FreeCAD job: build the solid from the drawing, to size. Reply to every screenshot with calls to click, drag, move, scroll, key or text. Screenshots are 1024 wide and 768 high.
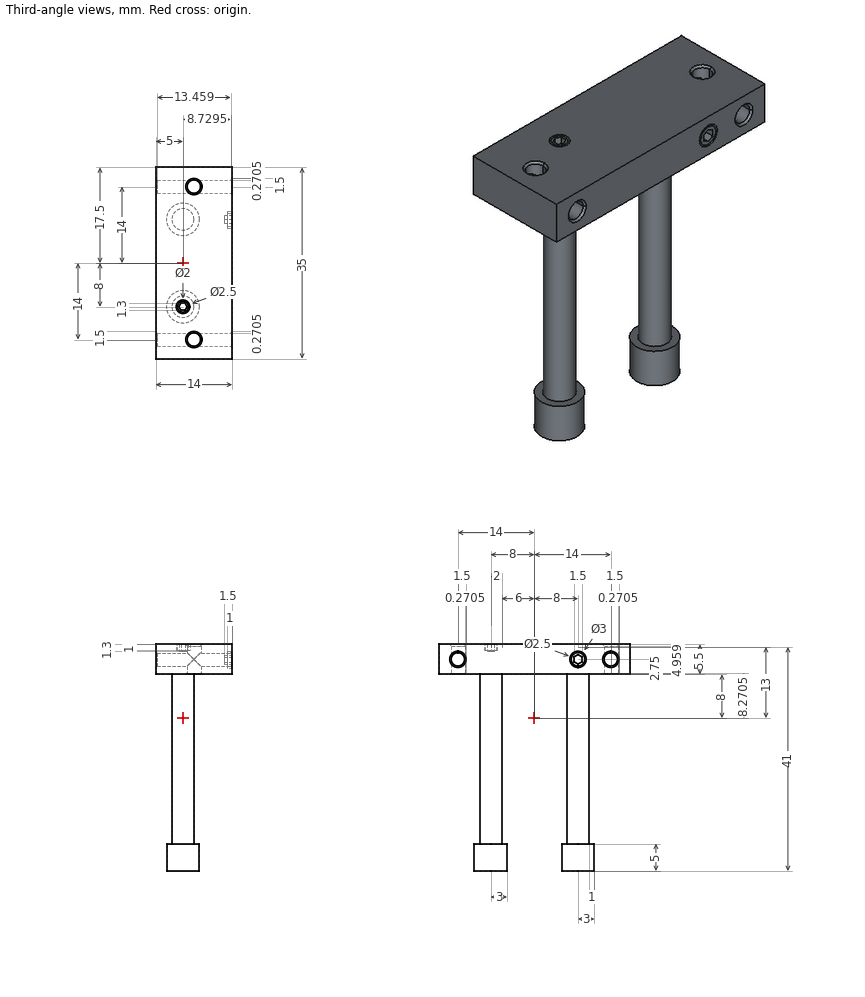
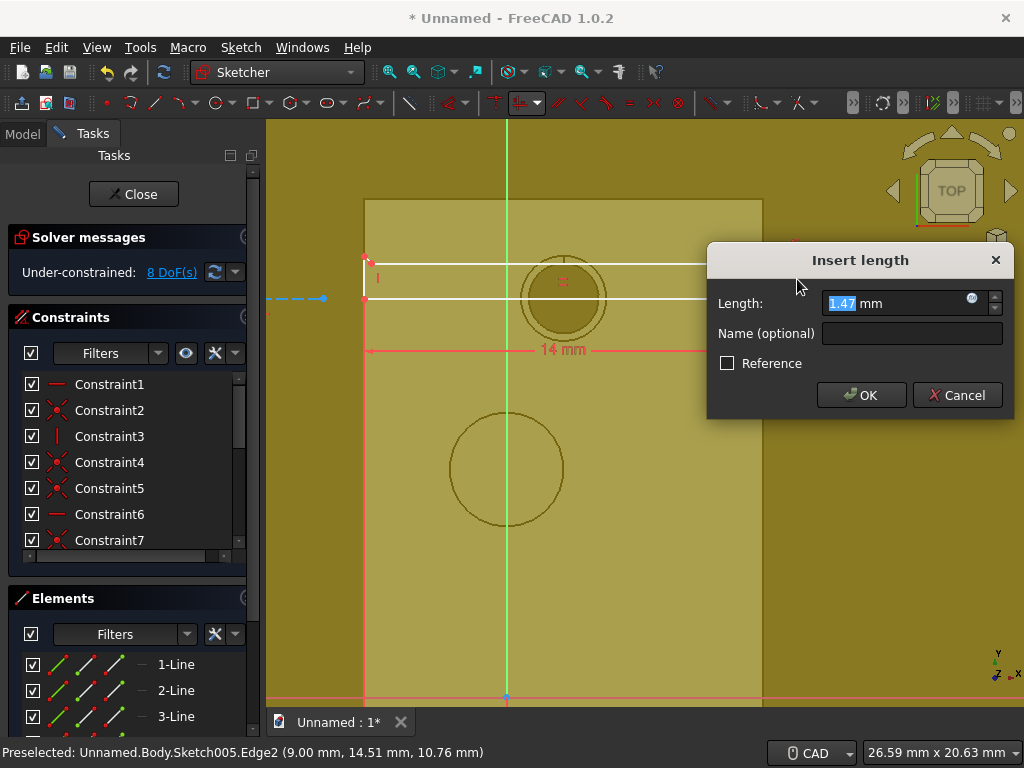
text(1.5)
key(Return)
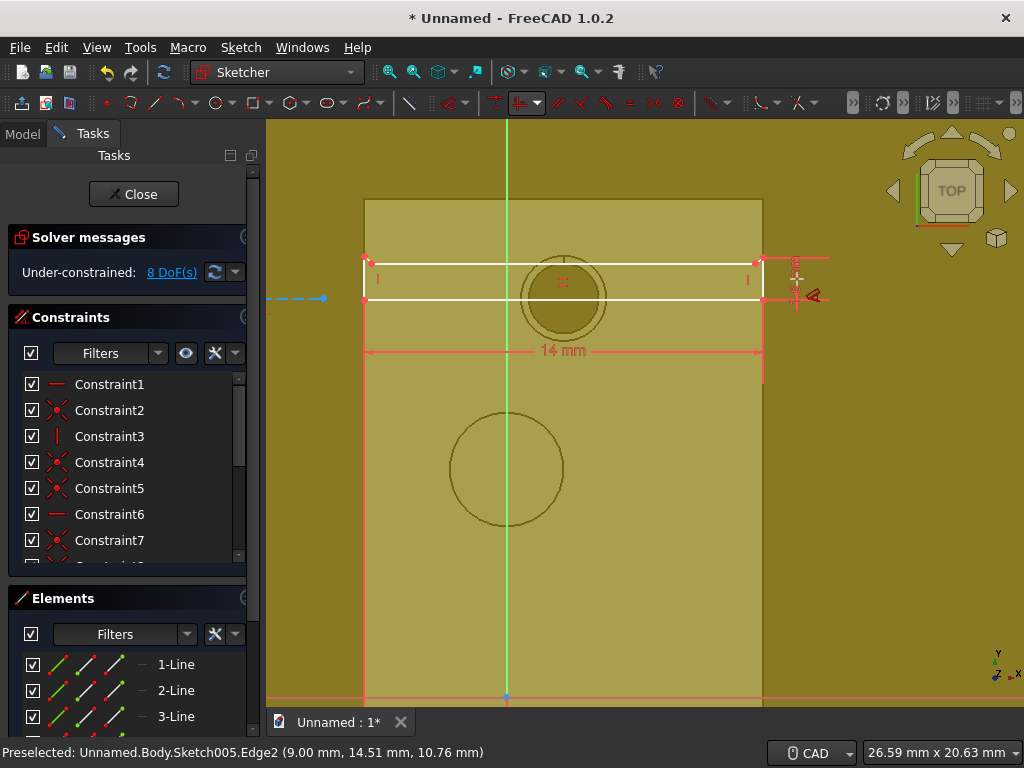
scroll(364, 269, up, 2)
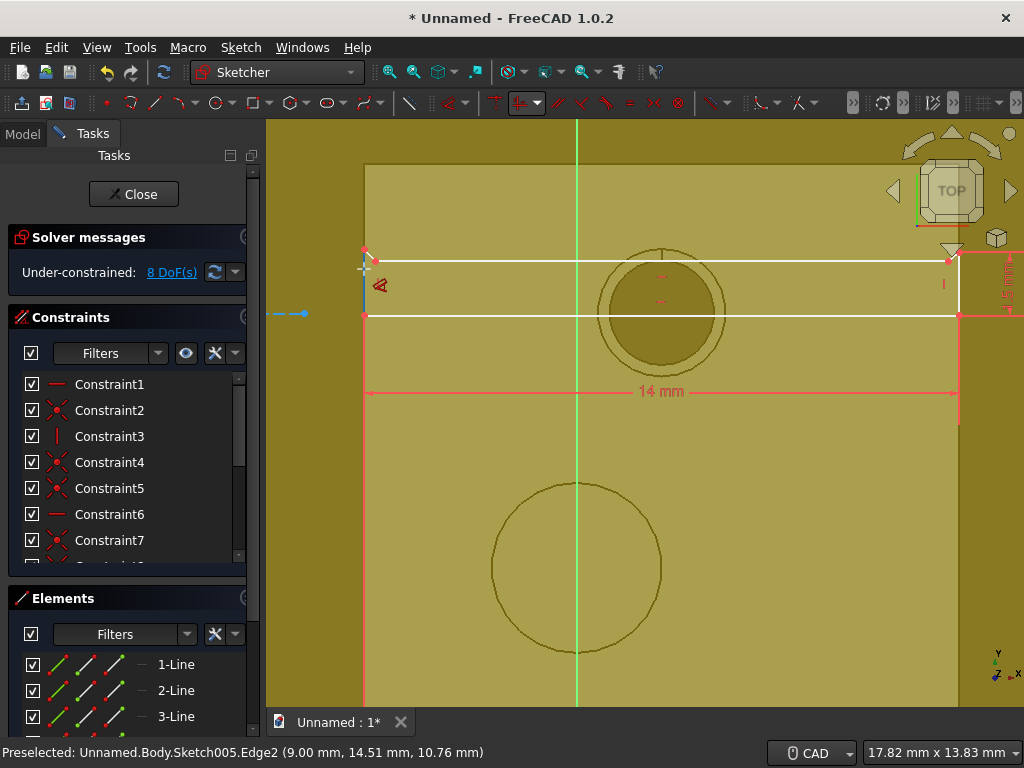
click(364, 269)
click(330, 283)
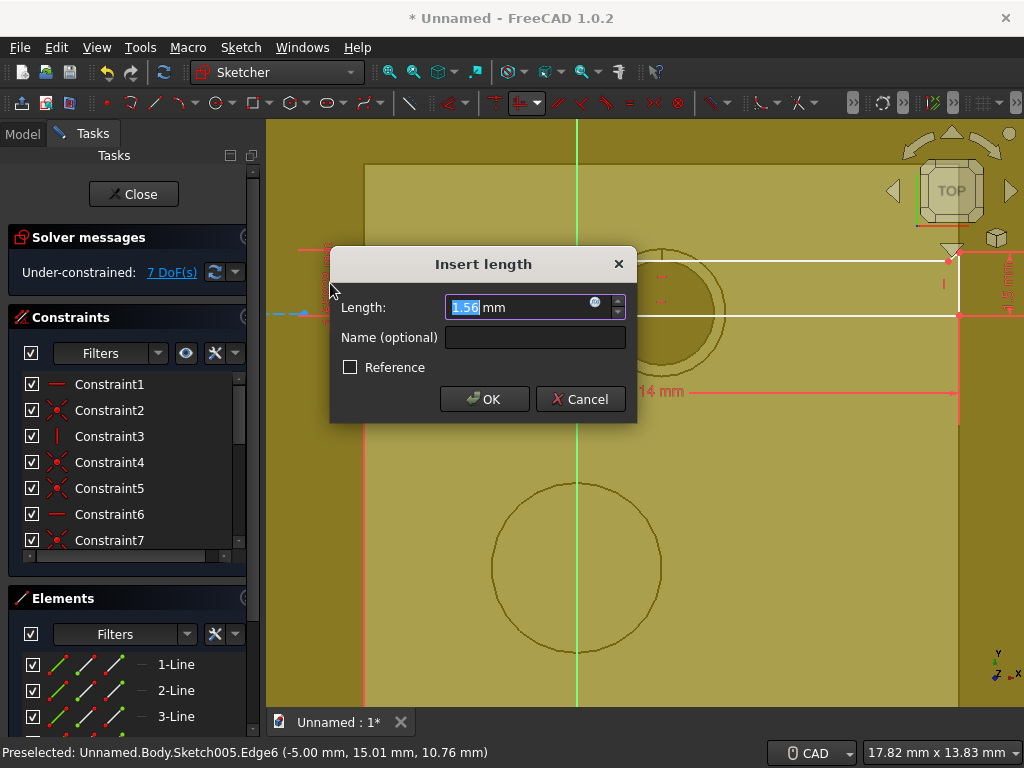
text(1.5)
key(Return)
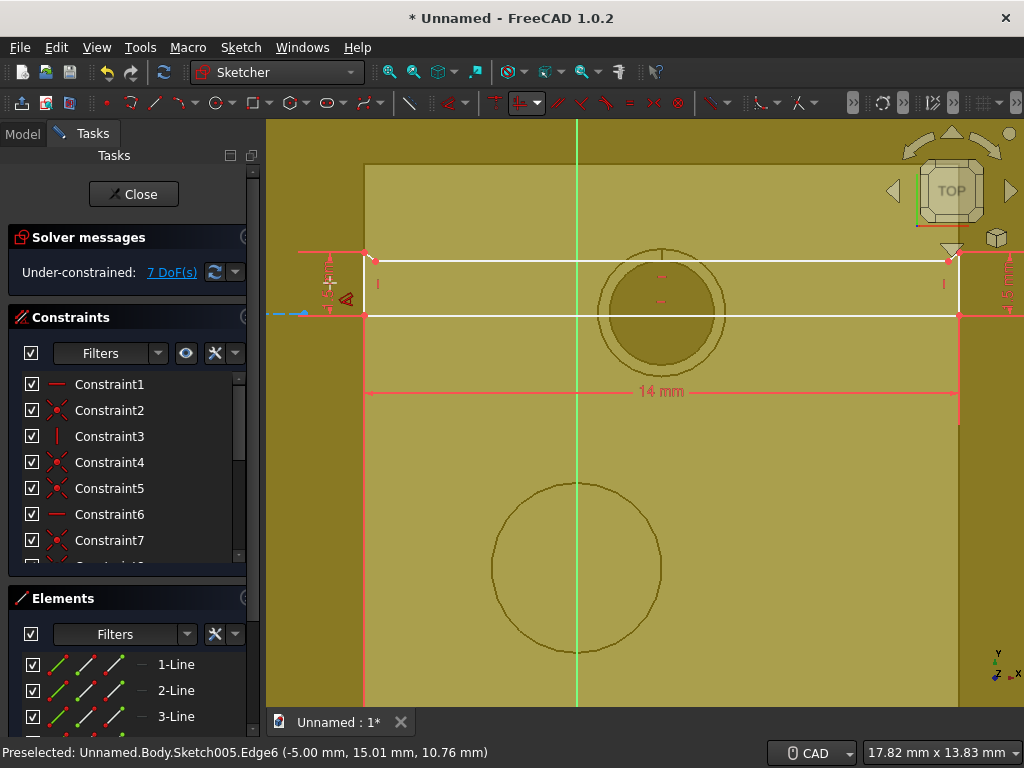
click(364, 316)
click(330, 497)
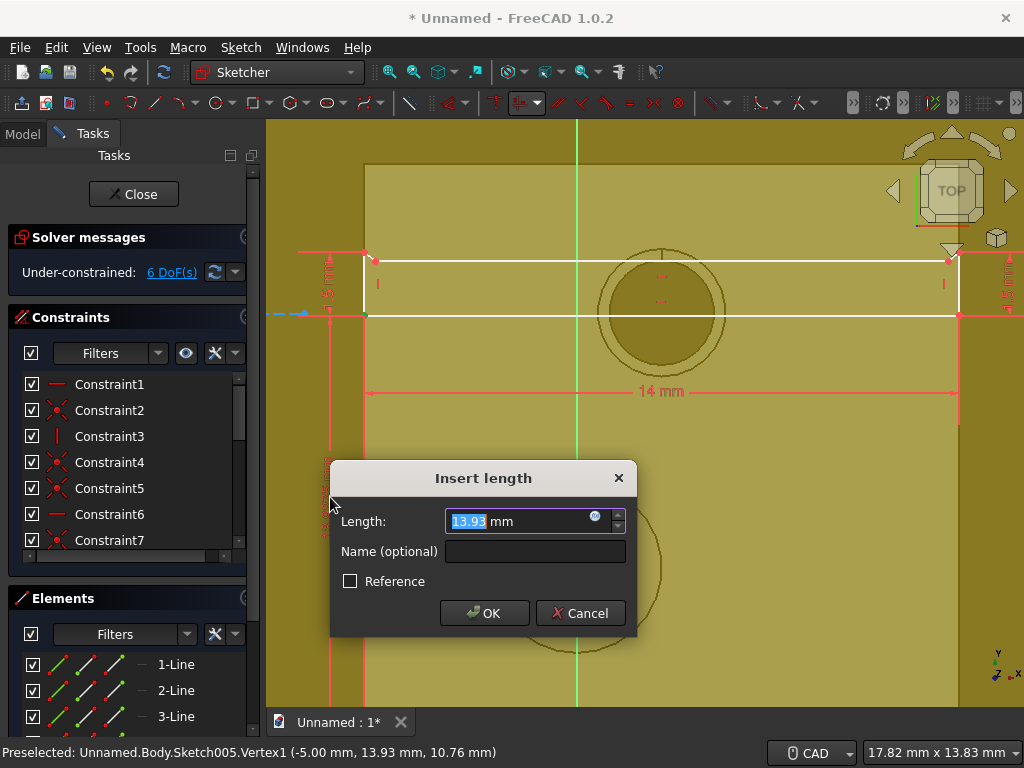
text(14)
key(Return)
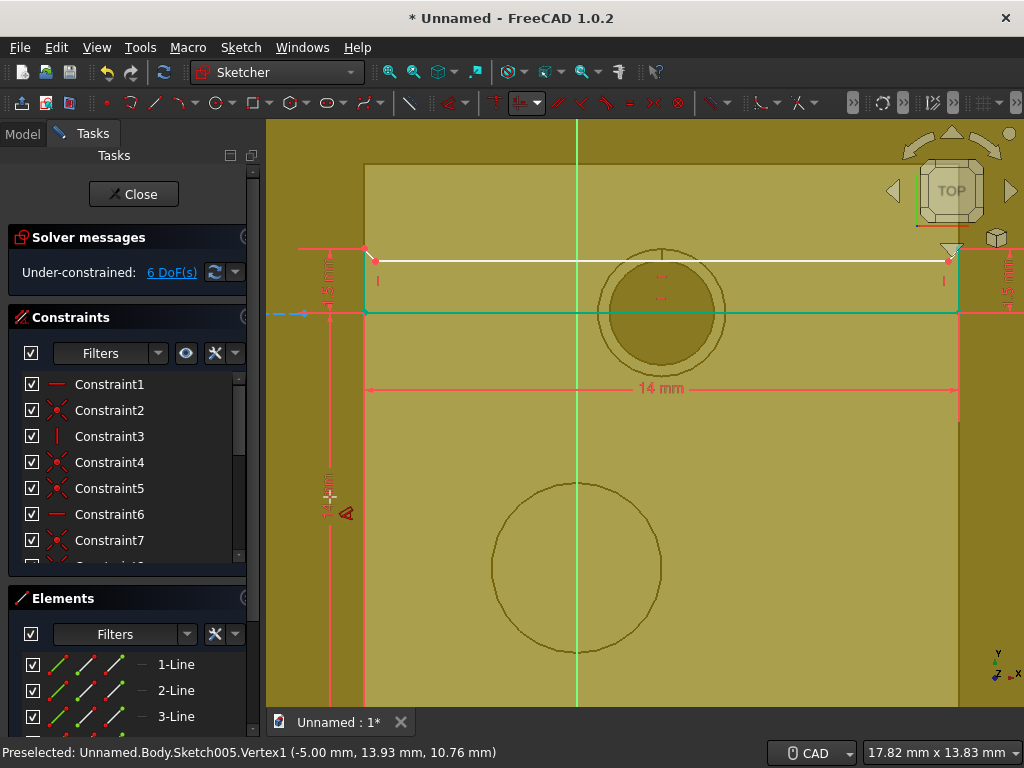
click(304, 314)
click(611, 496)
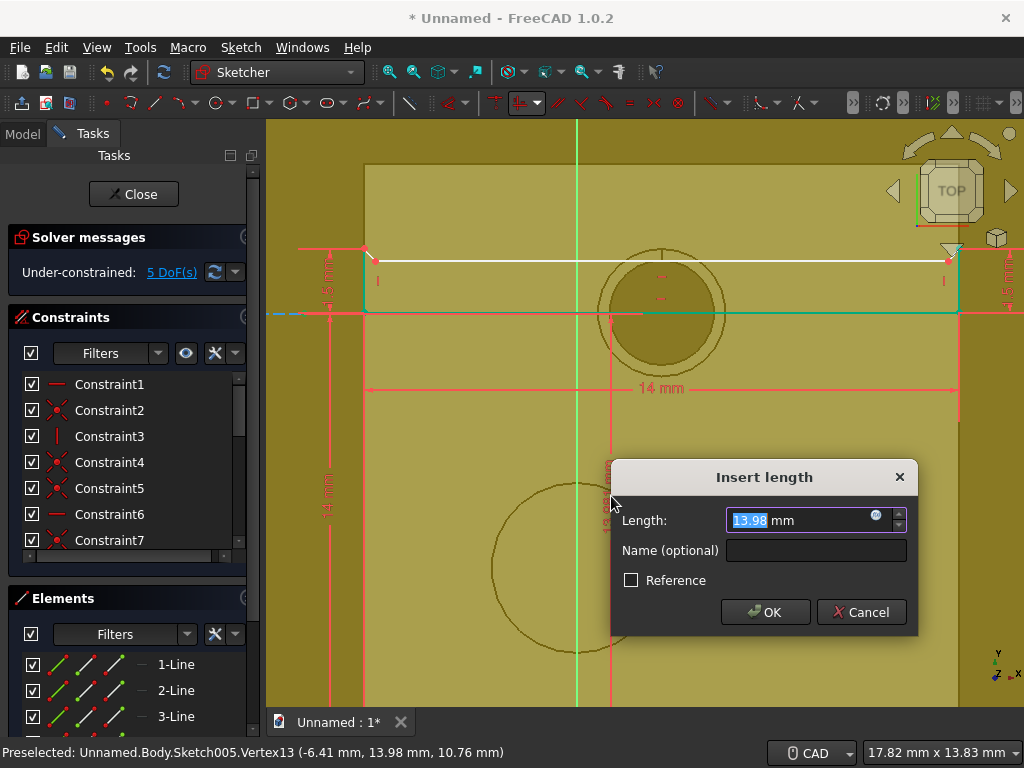
text(14)
key(Return)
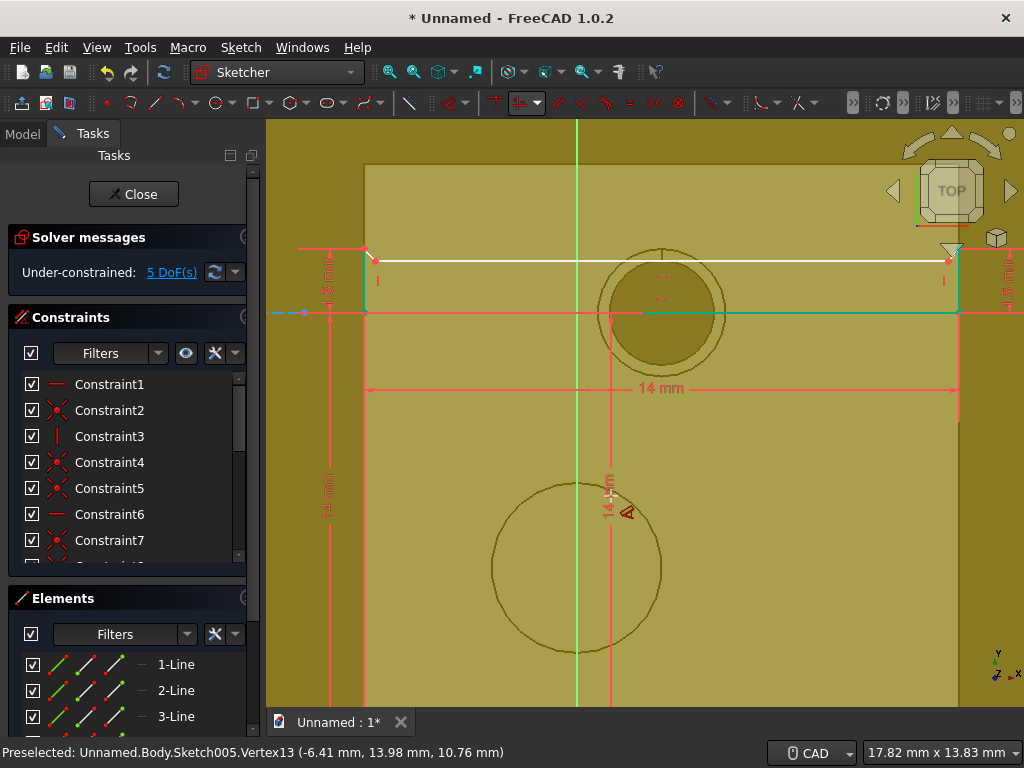
click(776, 261)
click(617, 227)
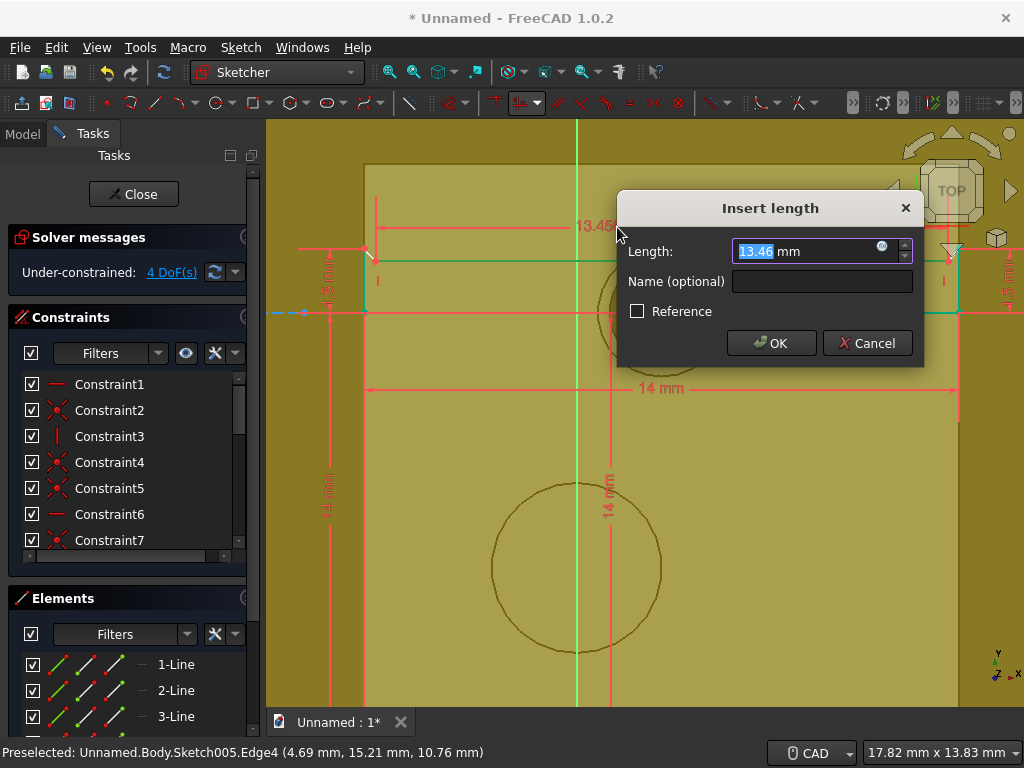
text(13.459)
key(Return)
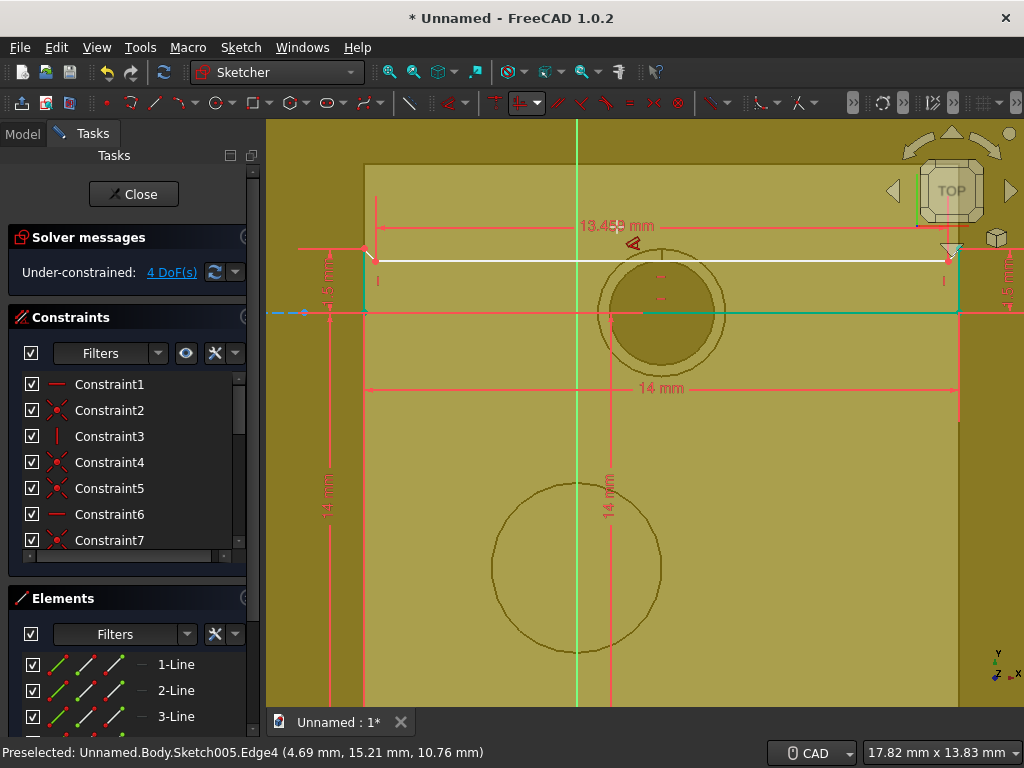
scroll(604, 278, down, 4)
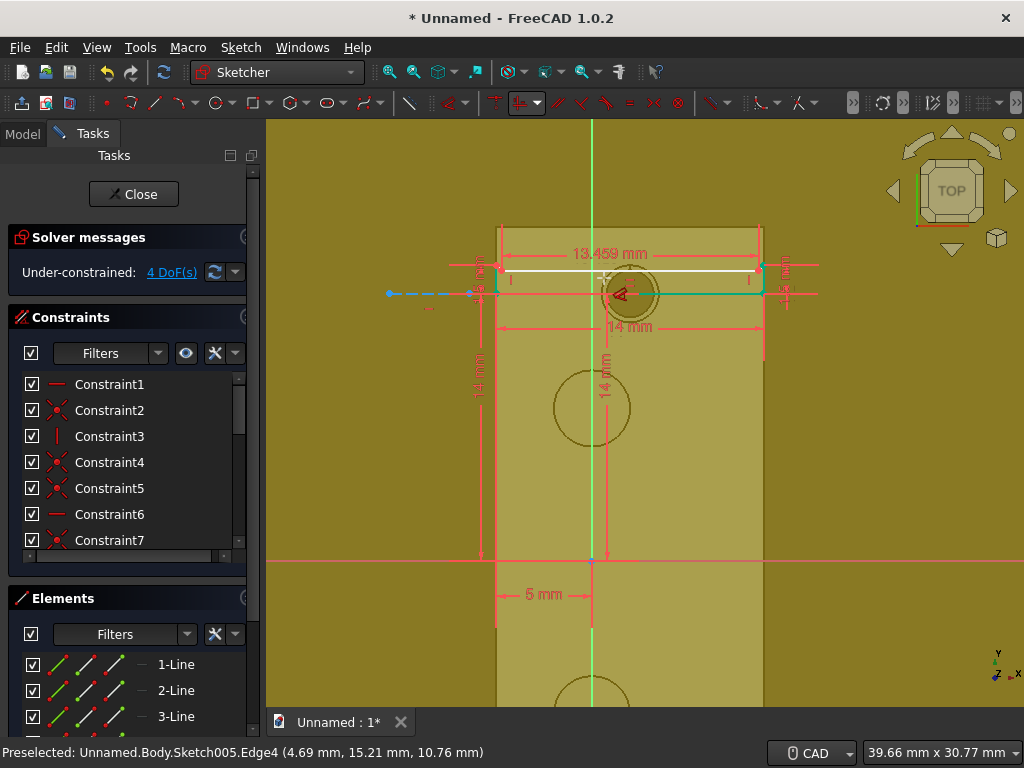
scroll(759, 271, up, 3)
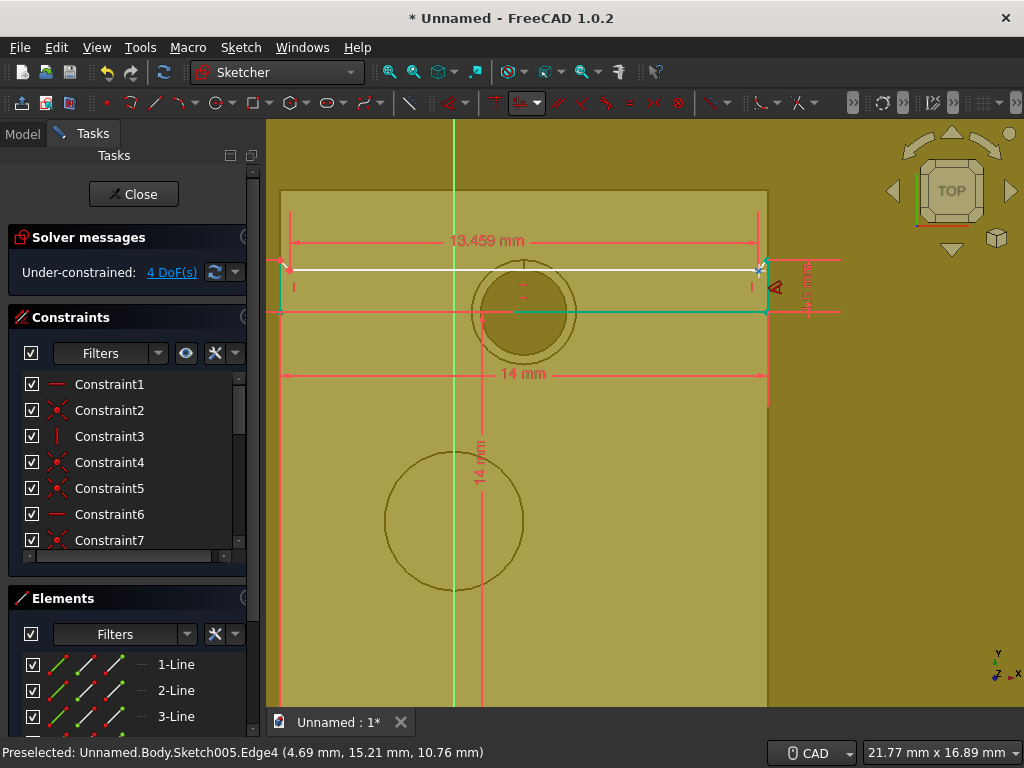
click(758, 270)
click(606, 236)